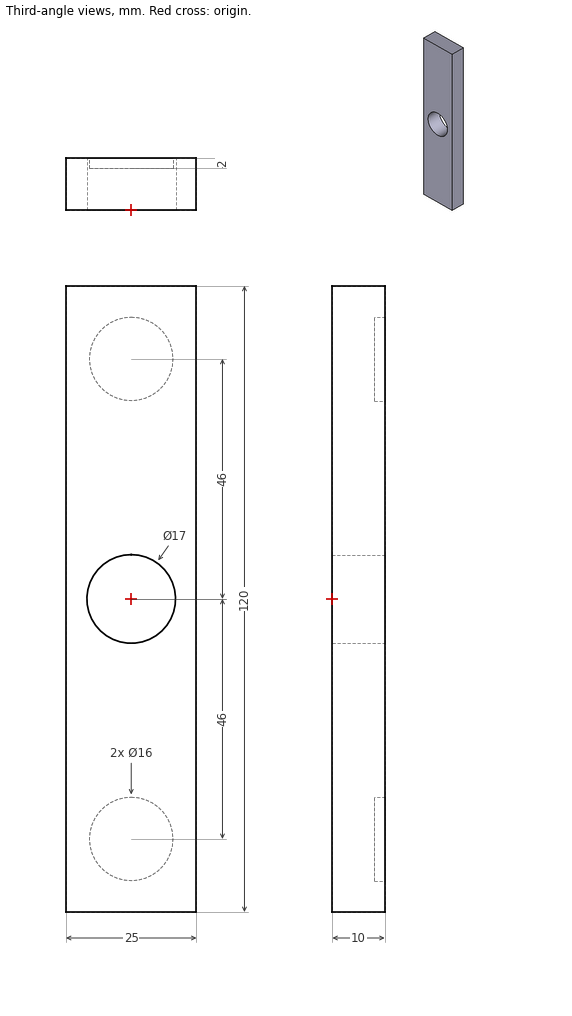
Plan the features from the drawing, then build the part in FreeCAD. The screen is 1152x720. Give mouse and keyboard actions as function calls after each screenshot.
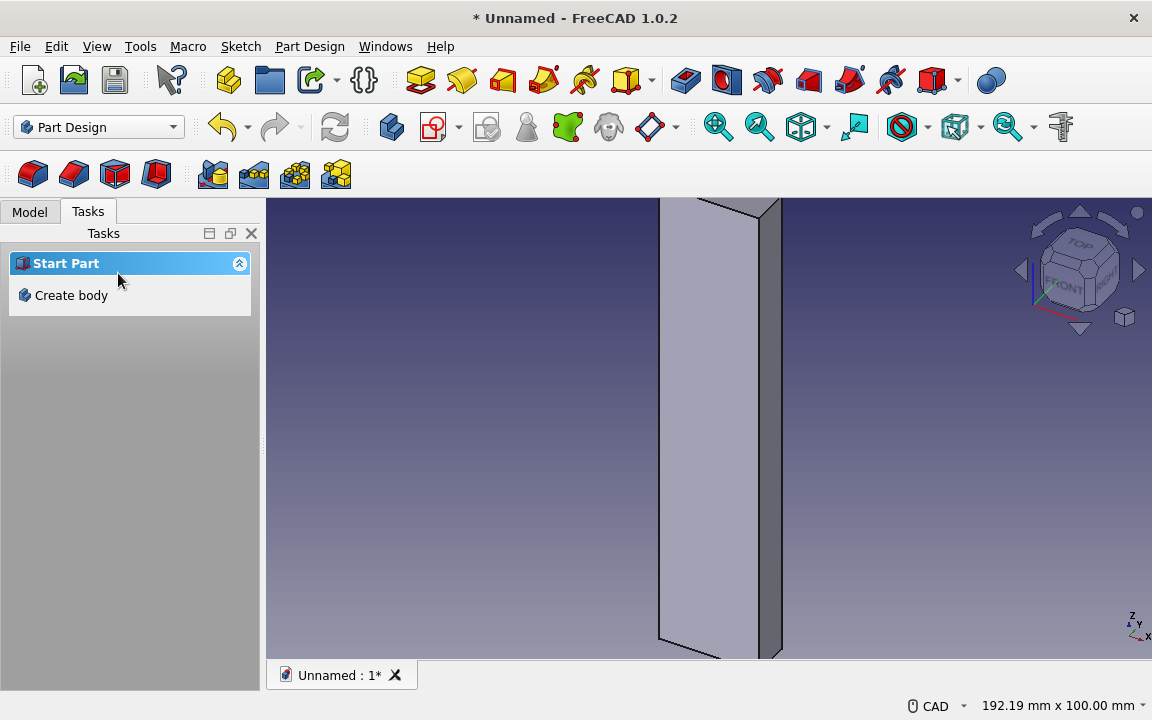
click(719, 128)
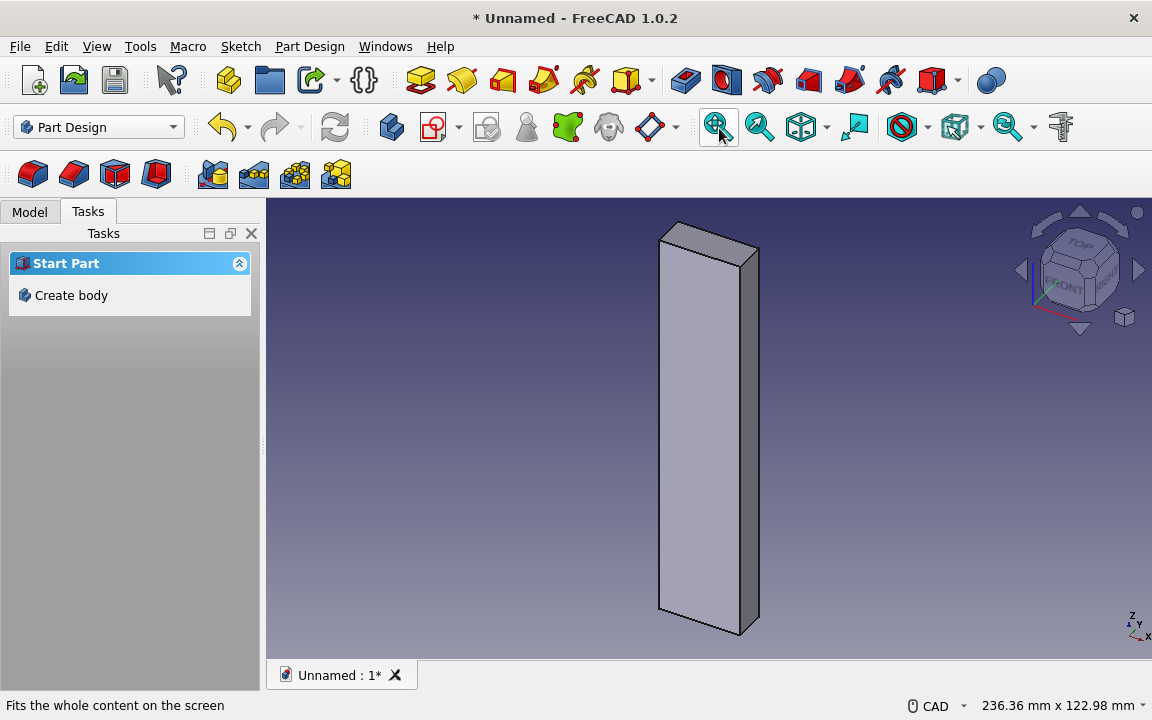
key(4)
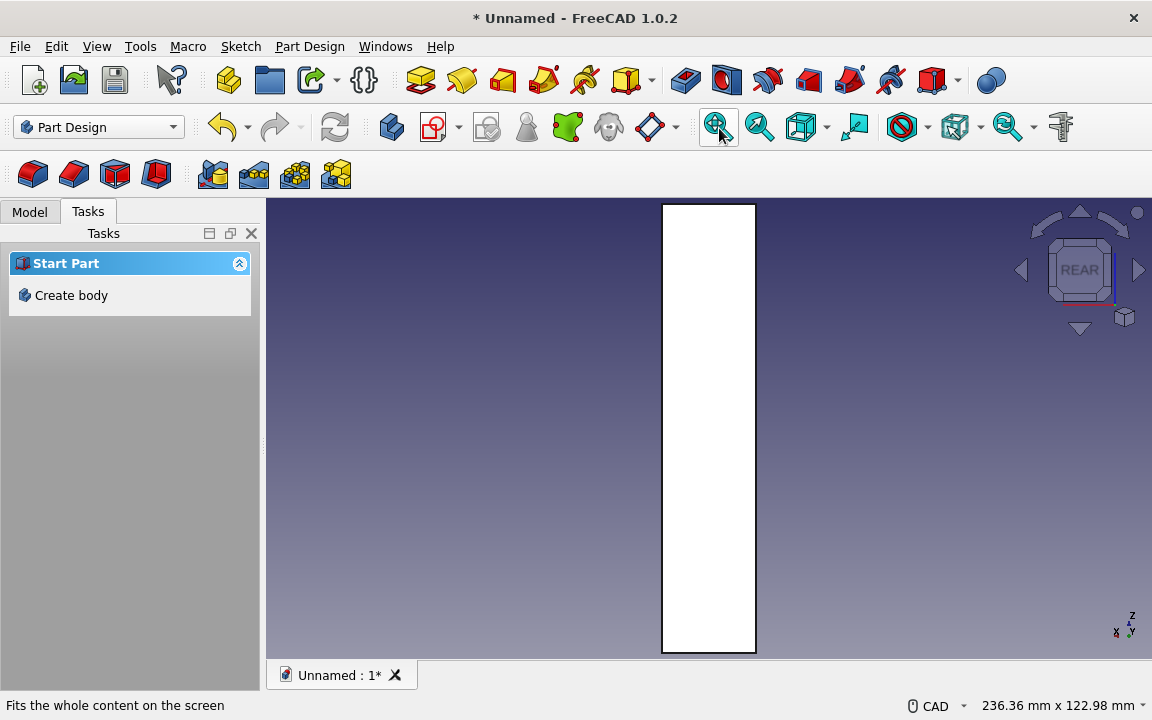
click(709, 299)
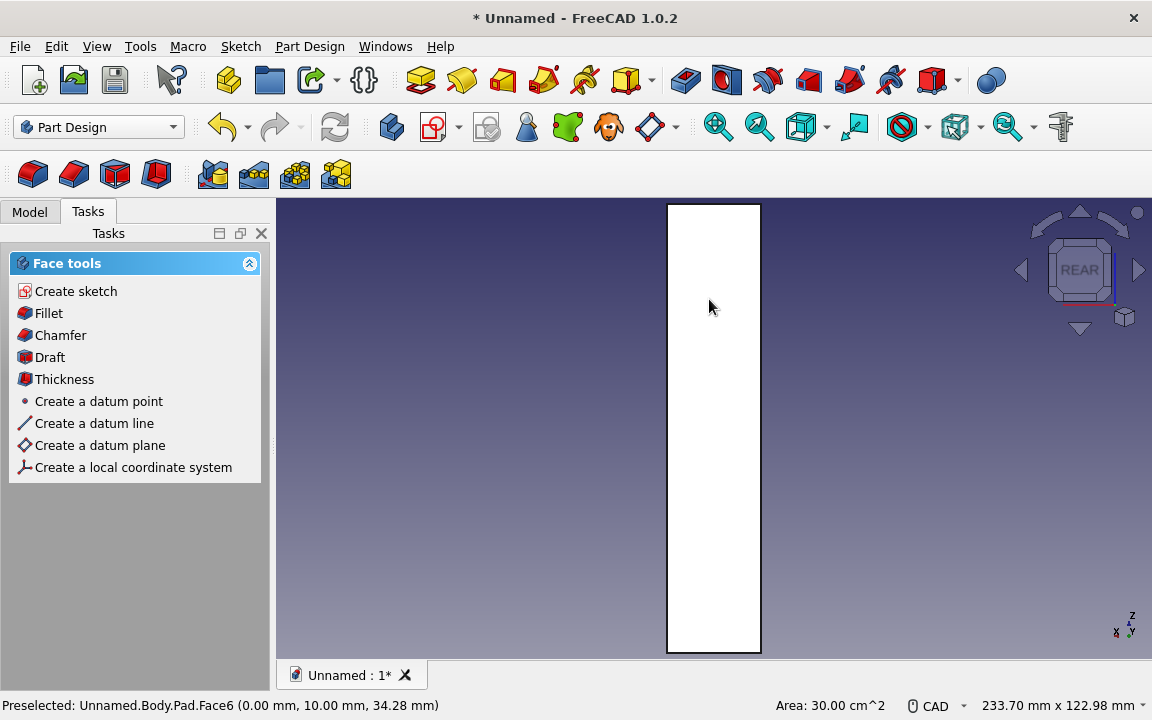
click(432, 128)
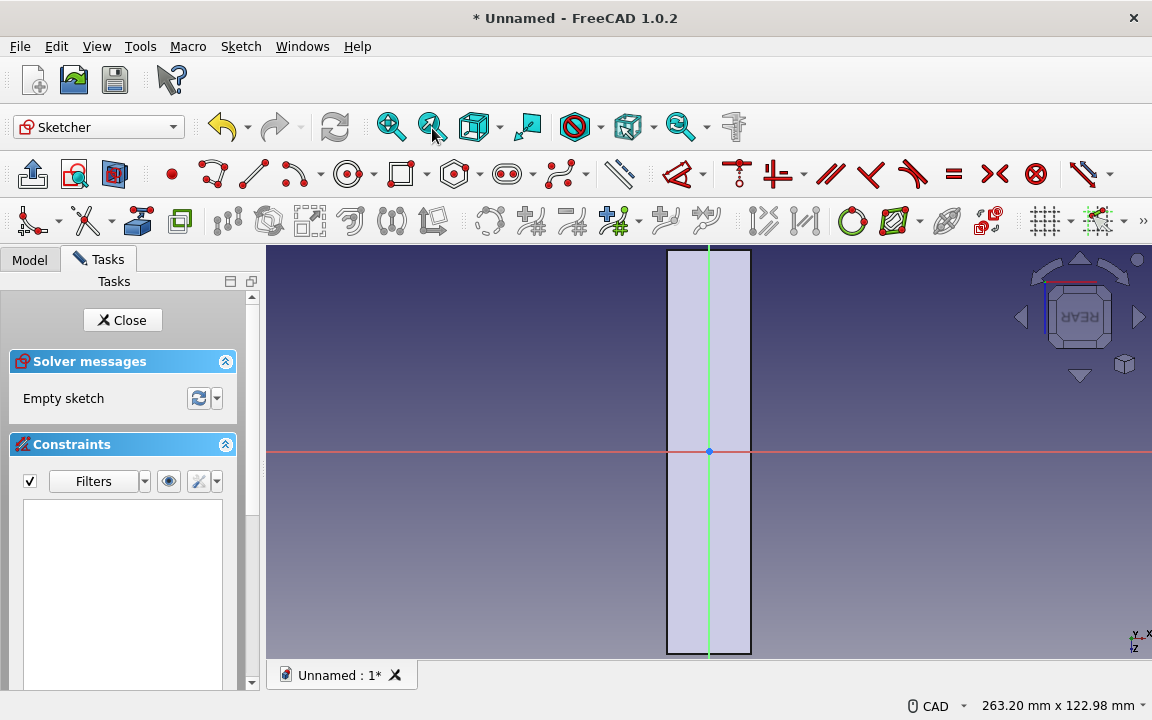
scroll(501, 452, down, 2)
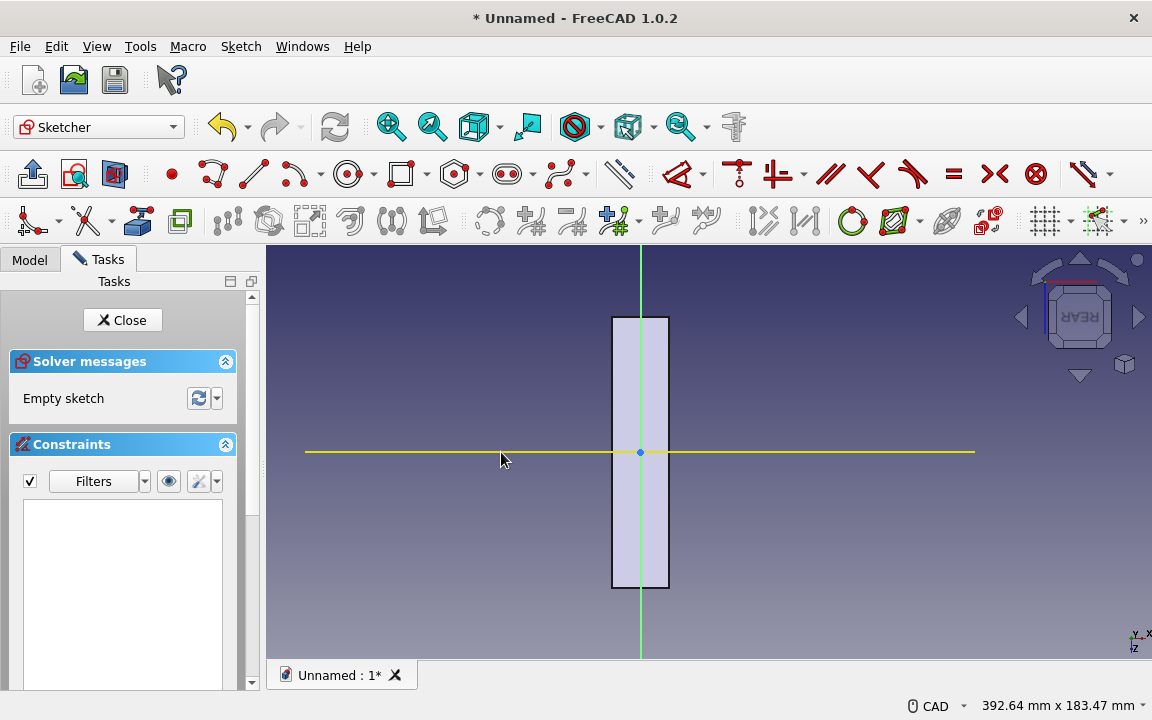
click(348, 174)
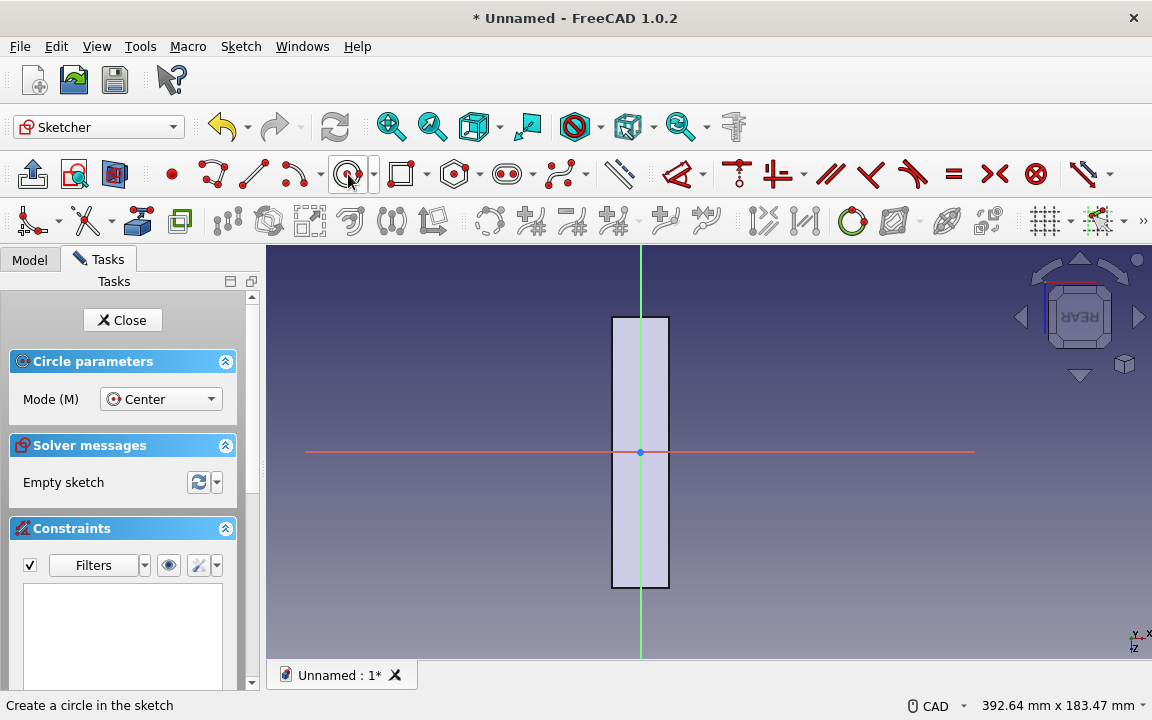
scroll(641, 348, up, 2)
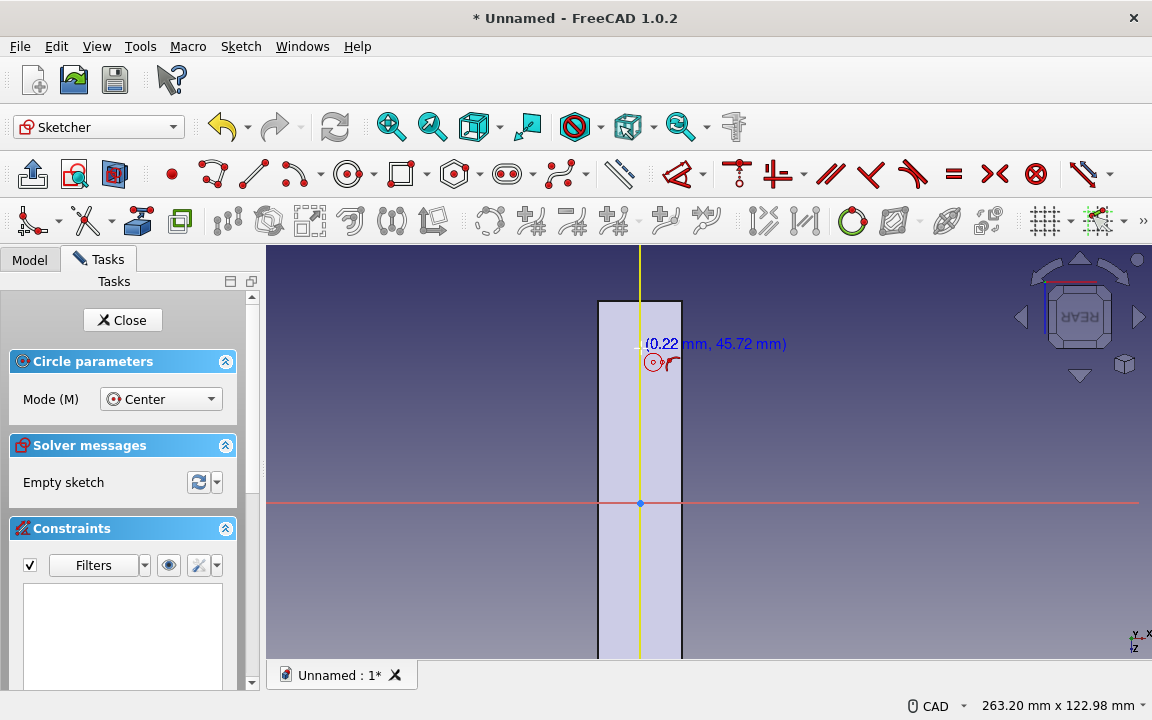
click(640, 348)
move(659, 329)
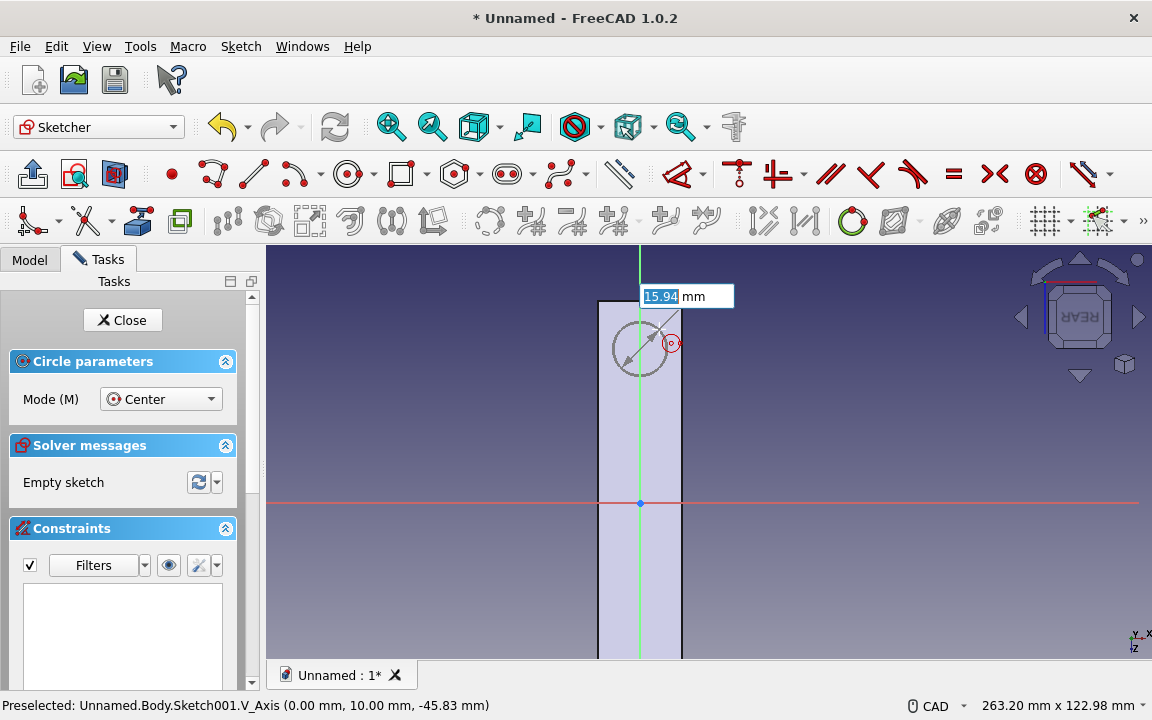
text(16)
key(Return)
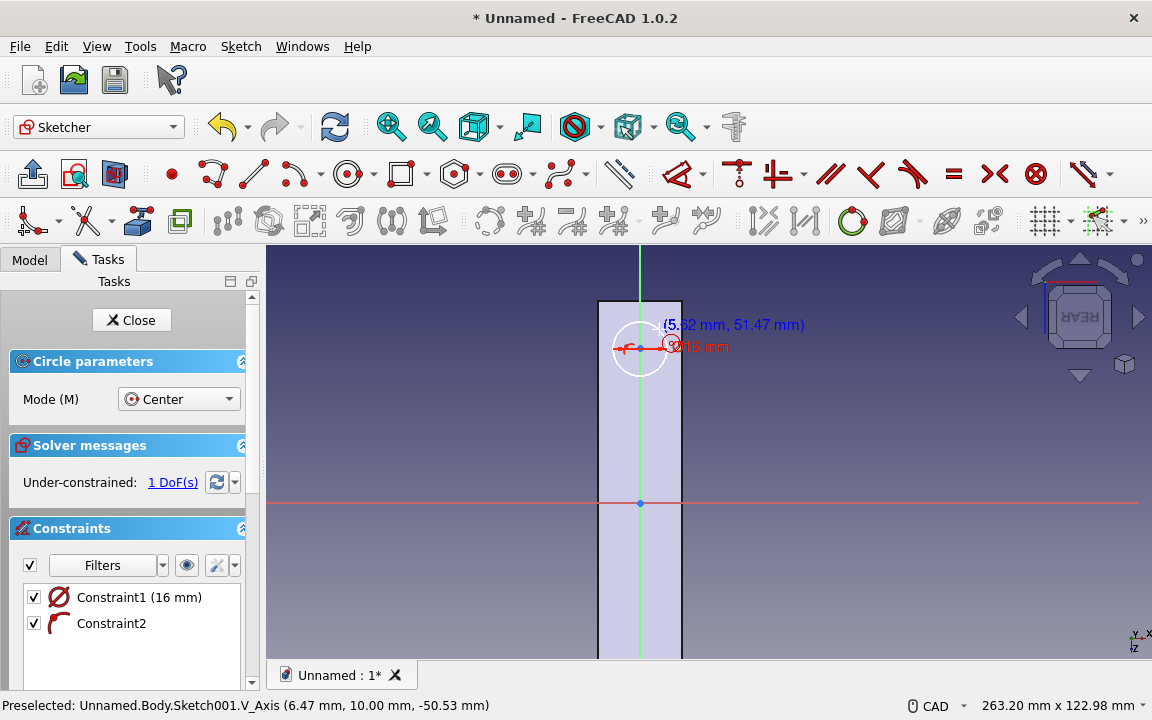
scroll(641, 348, down, 2)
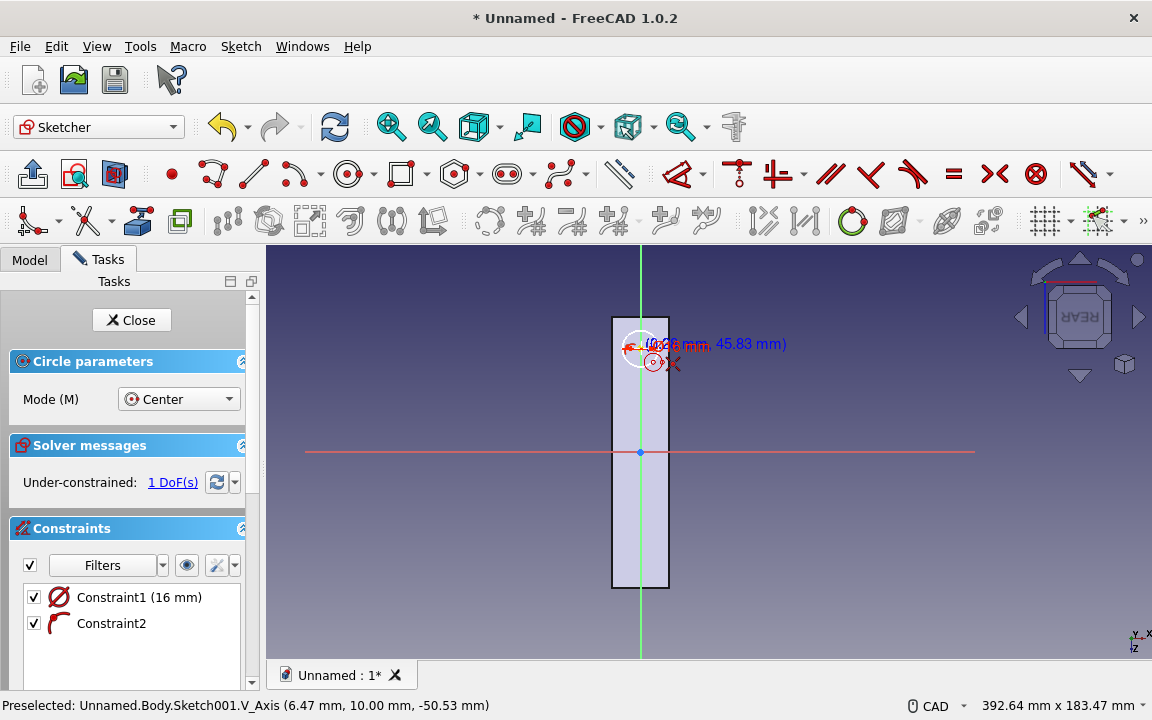
scroll(641, 556, up, 2)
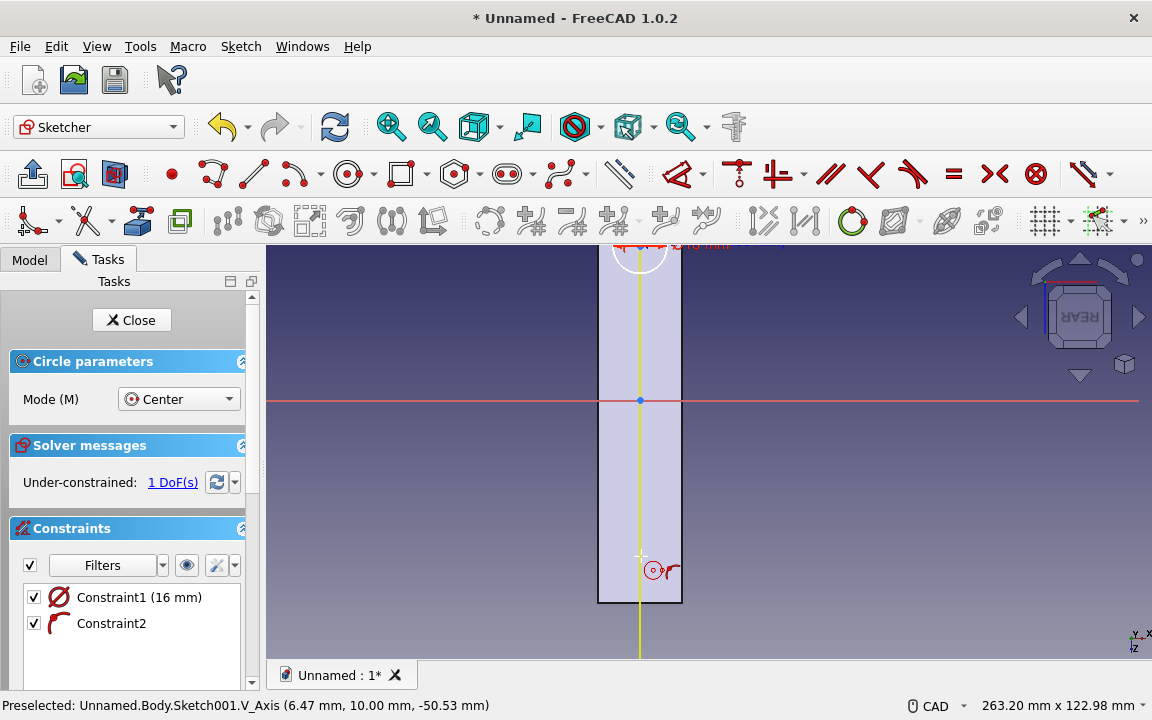
click(640, 556)
move(659, 537)